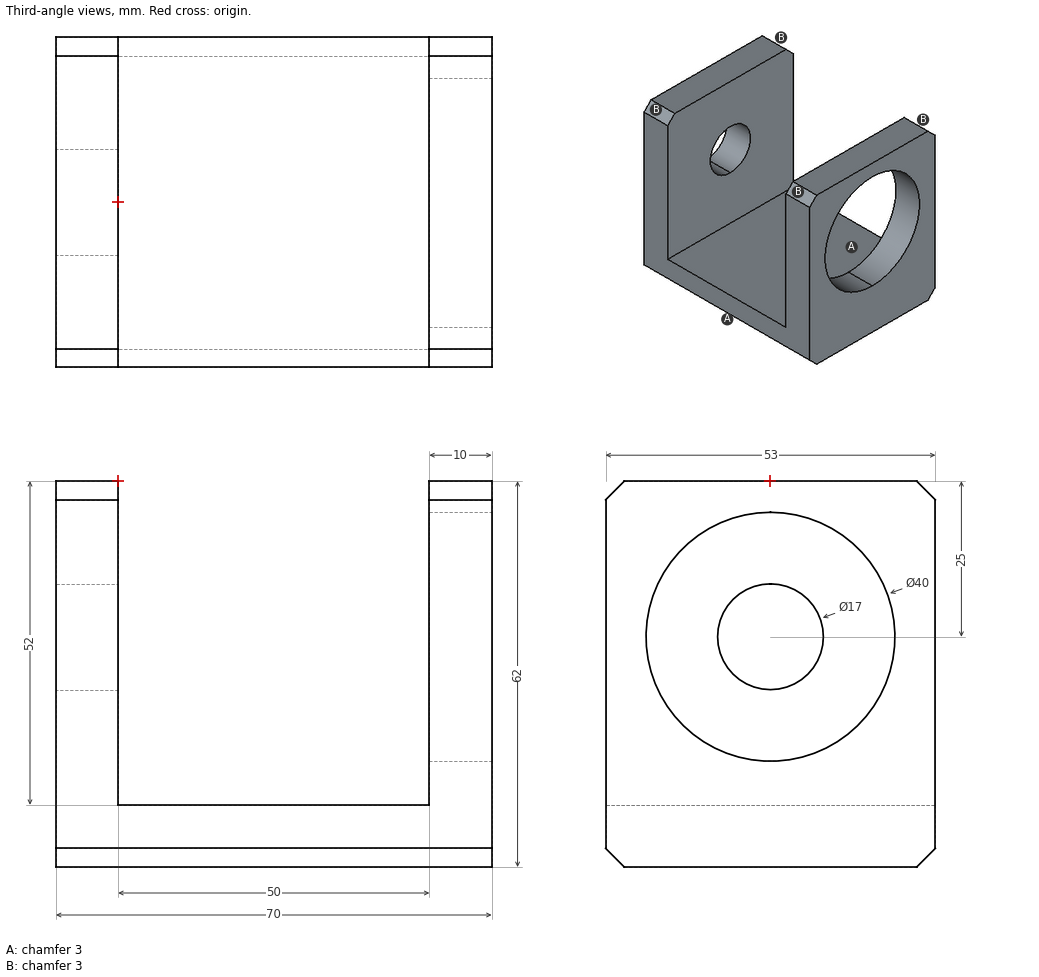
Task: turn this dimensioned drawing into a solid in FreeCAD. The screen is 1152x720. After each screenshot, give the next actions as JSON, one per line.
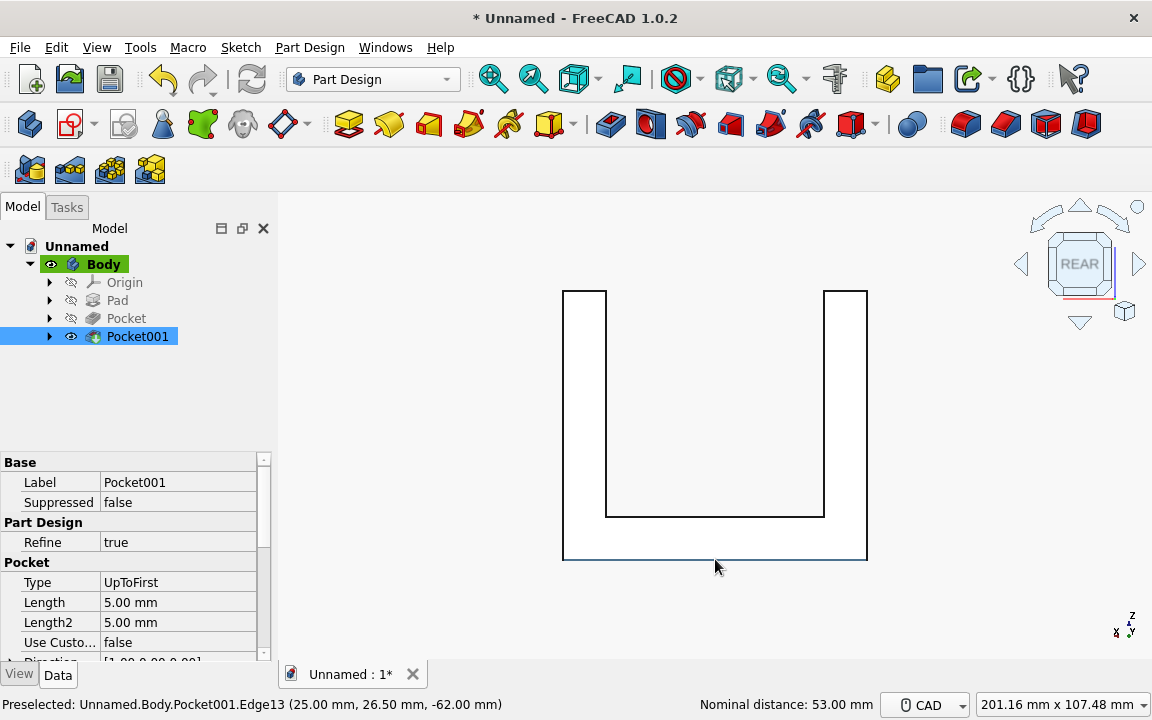
{"action": "left_click", "coordinate": [1006, 124]}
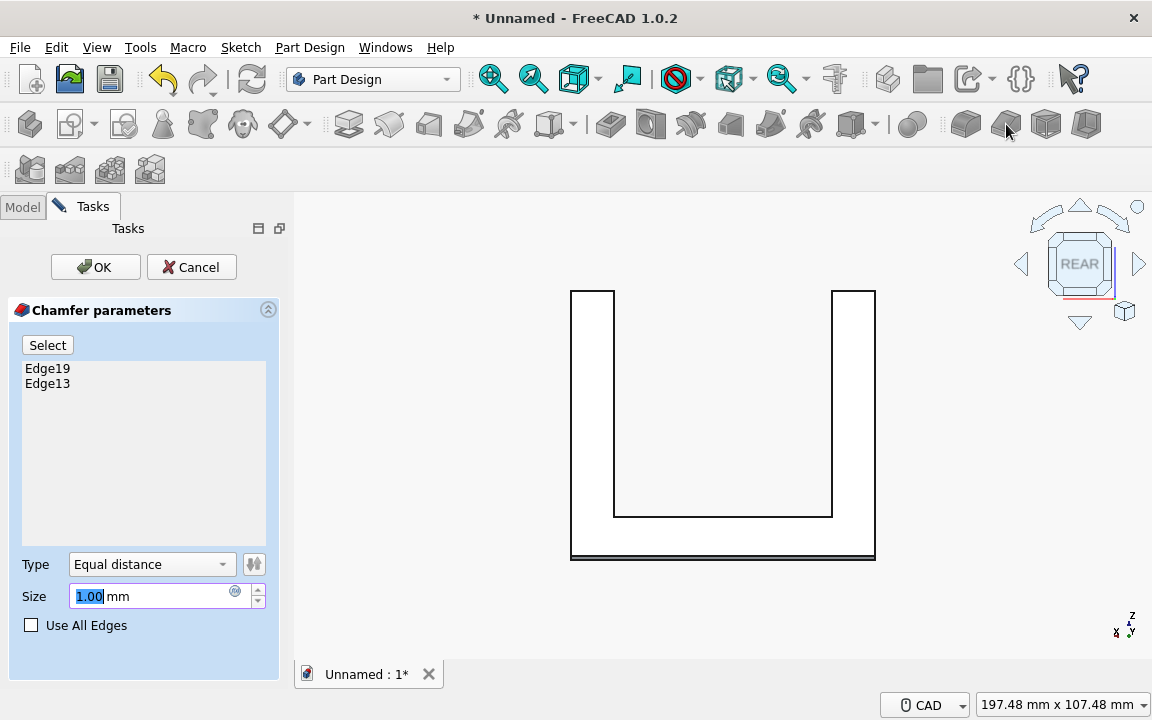
{"action": "type", "text": "3"}
{"action": "key", "text": "Tab"}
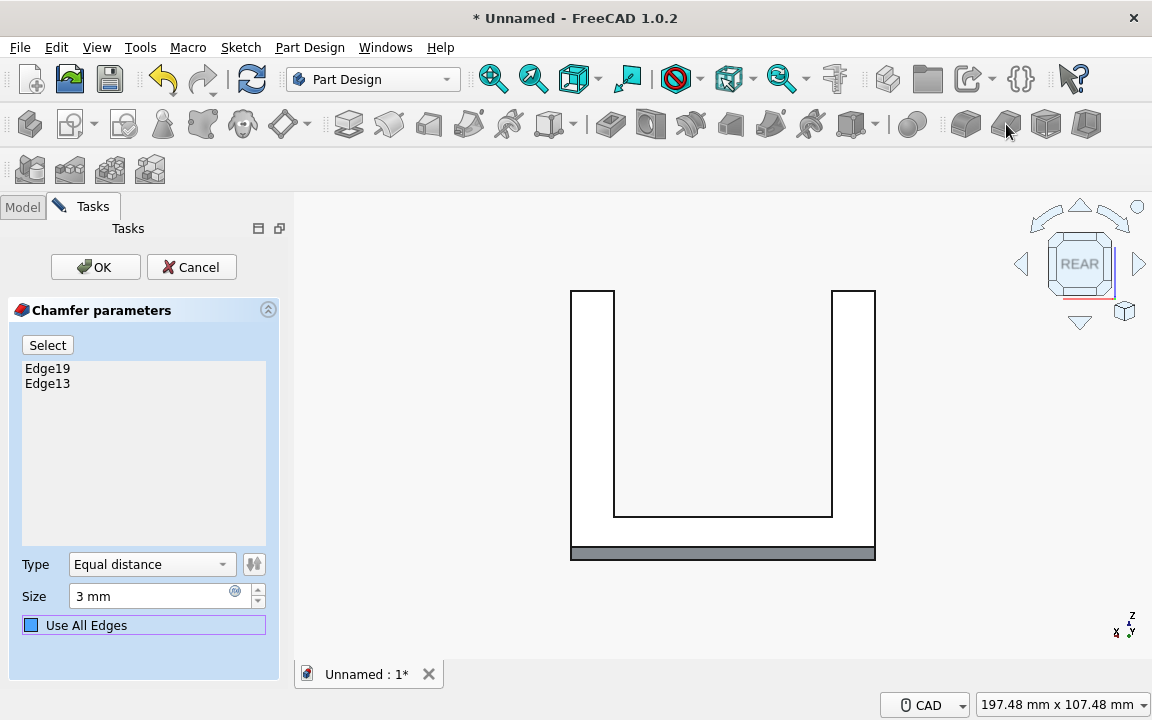
{"action": "left_click", "coordinate": [96, 267]}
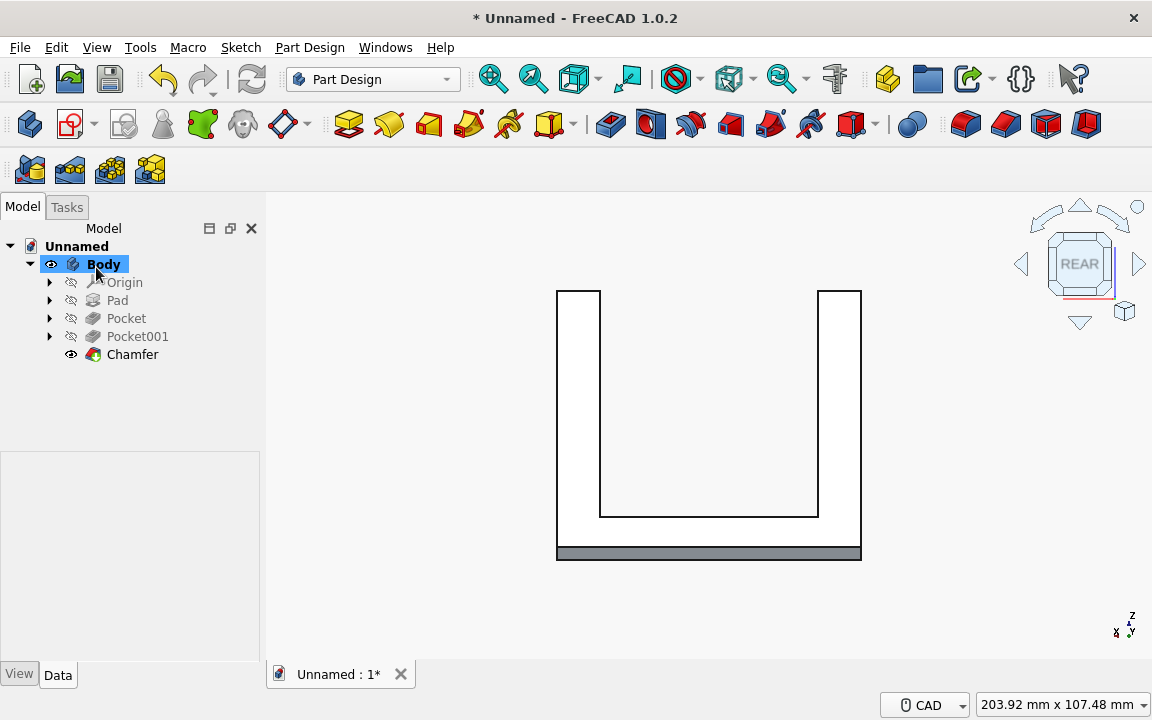
{"action": "key", "text": "0"}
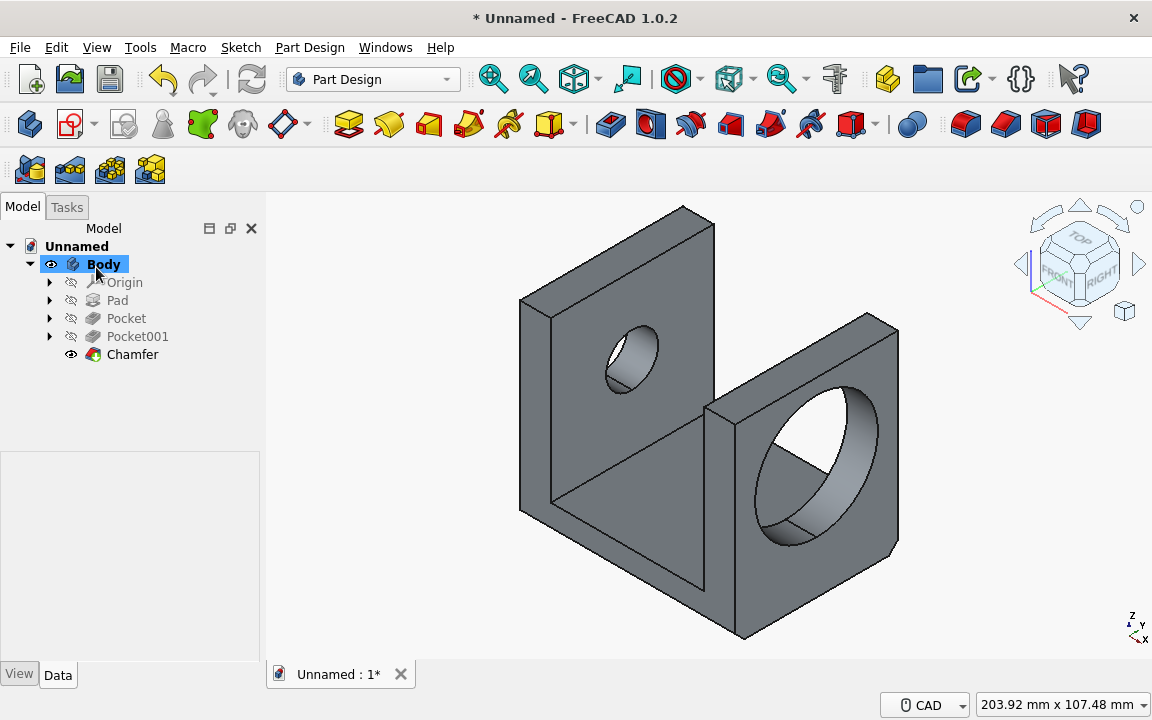
{"action": "left_click", "coordinate": [535, 308]}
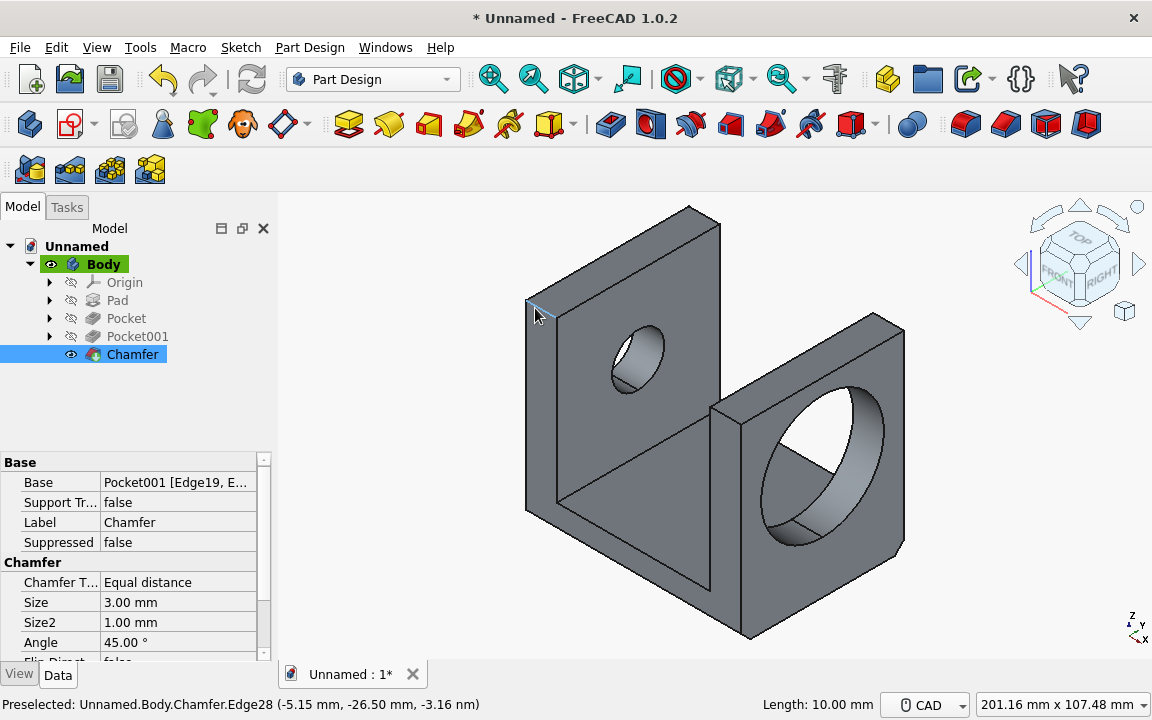
{"action": "left_click", "coordinate": [726, 415], "text": "ctrl"}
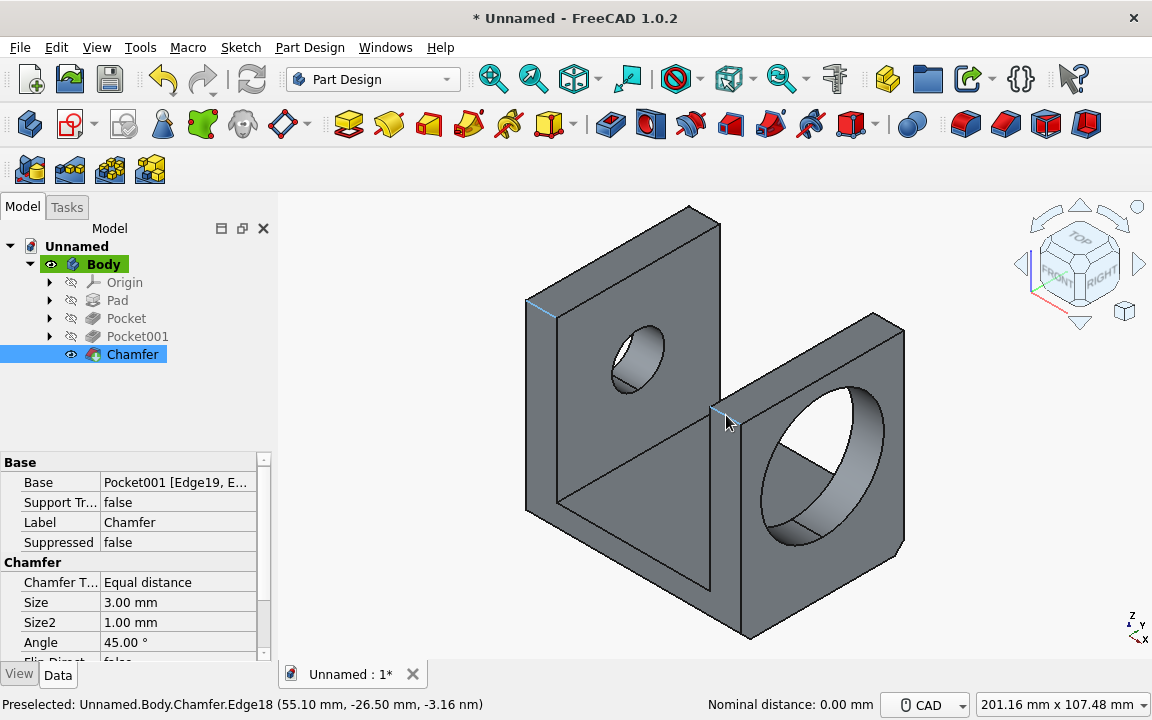
{"action": "key", "text": "2"}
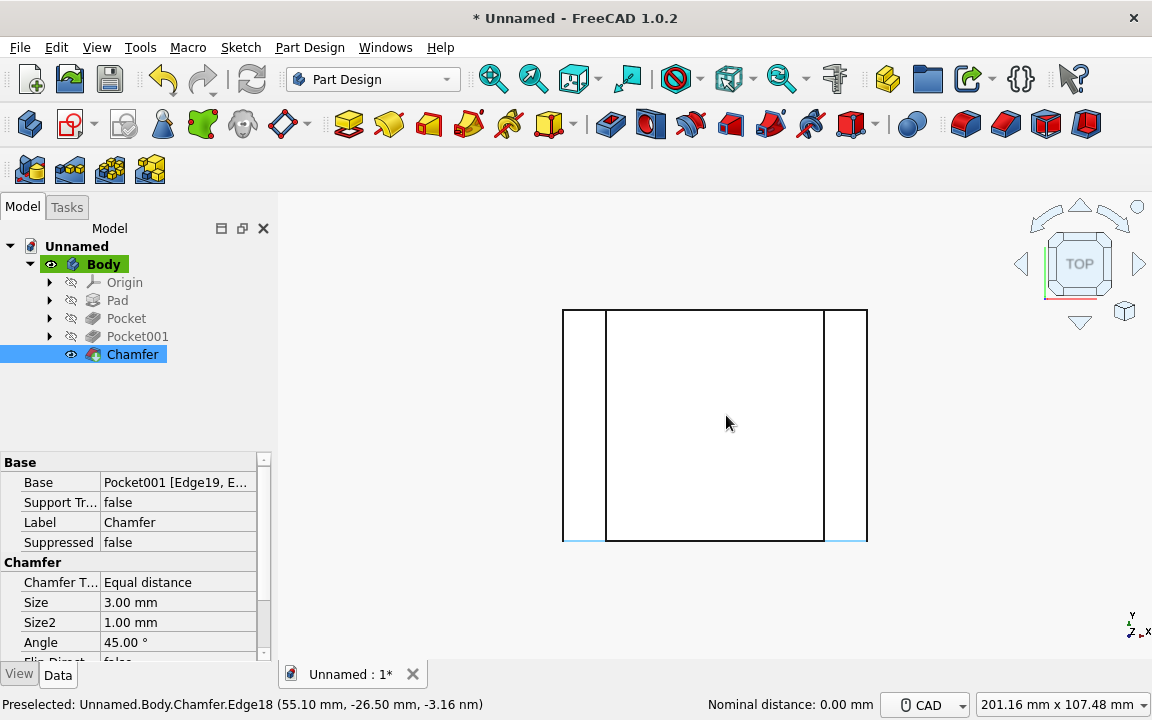
{"action": "left_click", "coordinate": [845, 309], "text": "ctrl"}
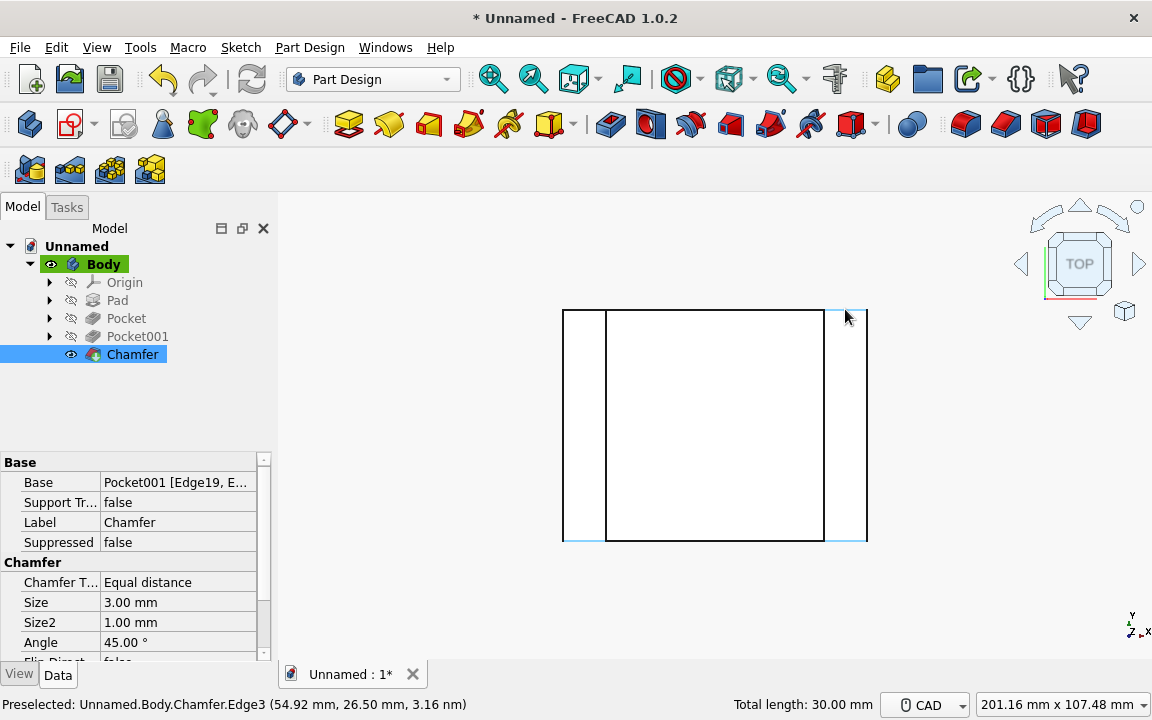
{"action": "left_click", "coordinate": [585, 309], "text": "ctrl"}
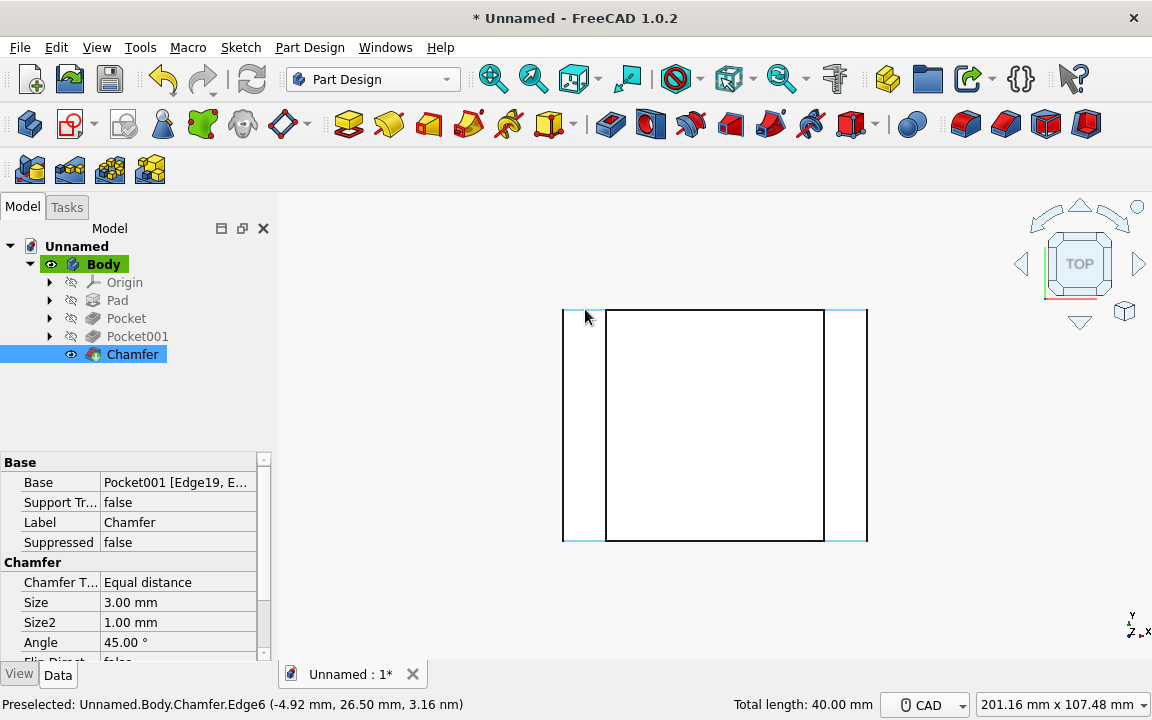
{"action": "left_click", "coordinate": [1006, 124]}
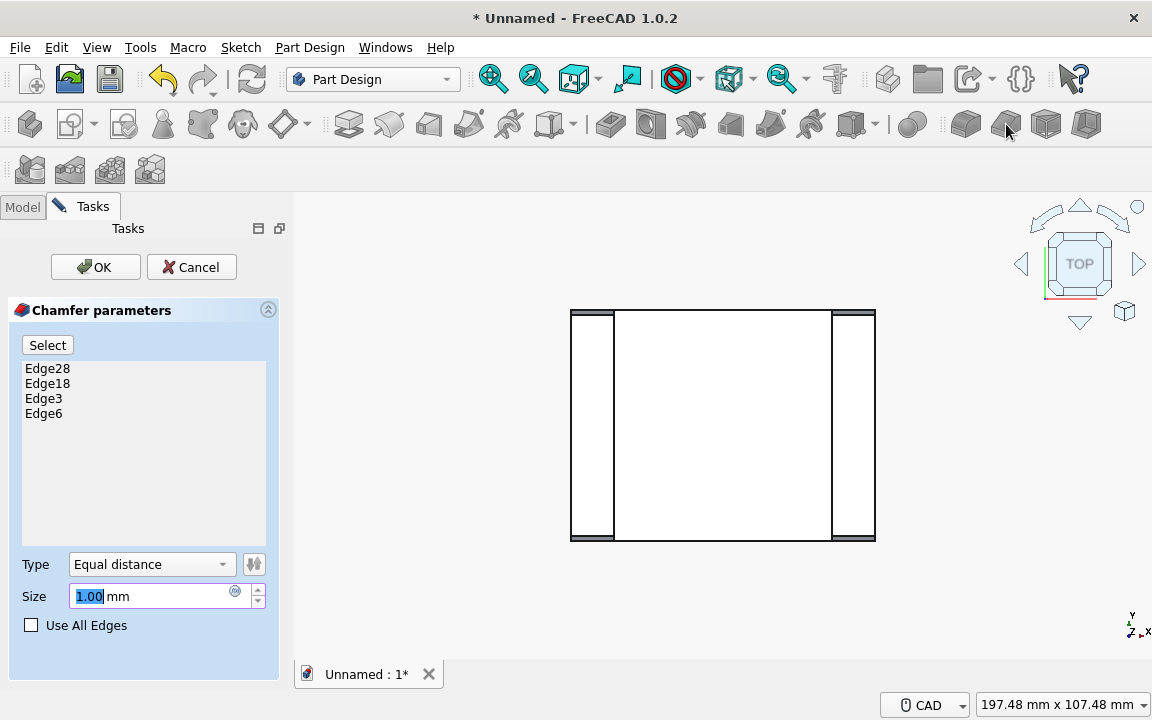
{"action": "type", "text": "3"}
{"action": "key", "text": "Tab"}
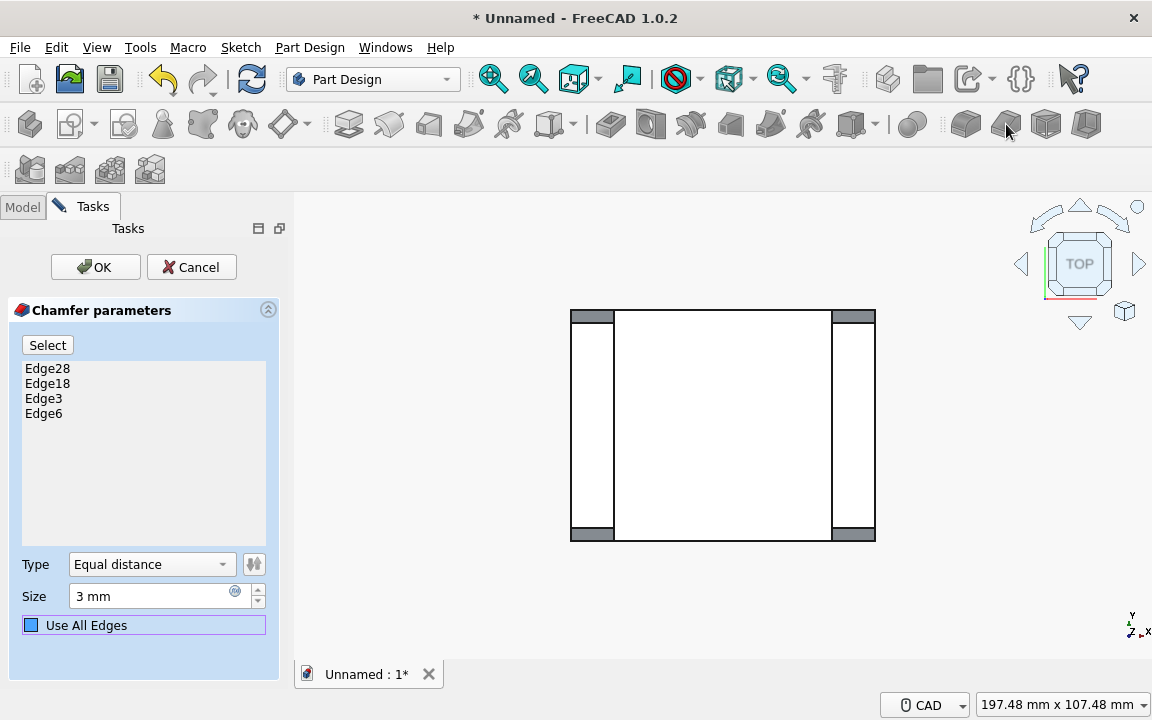
{"action": "left_click", "coordinate": [96, 267]}